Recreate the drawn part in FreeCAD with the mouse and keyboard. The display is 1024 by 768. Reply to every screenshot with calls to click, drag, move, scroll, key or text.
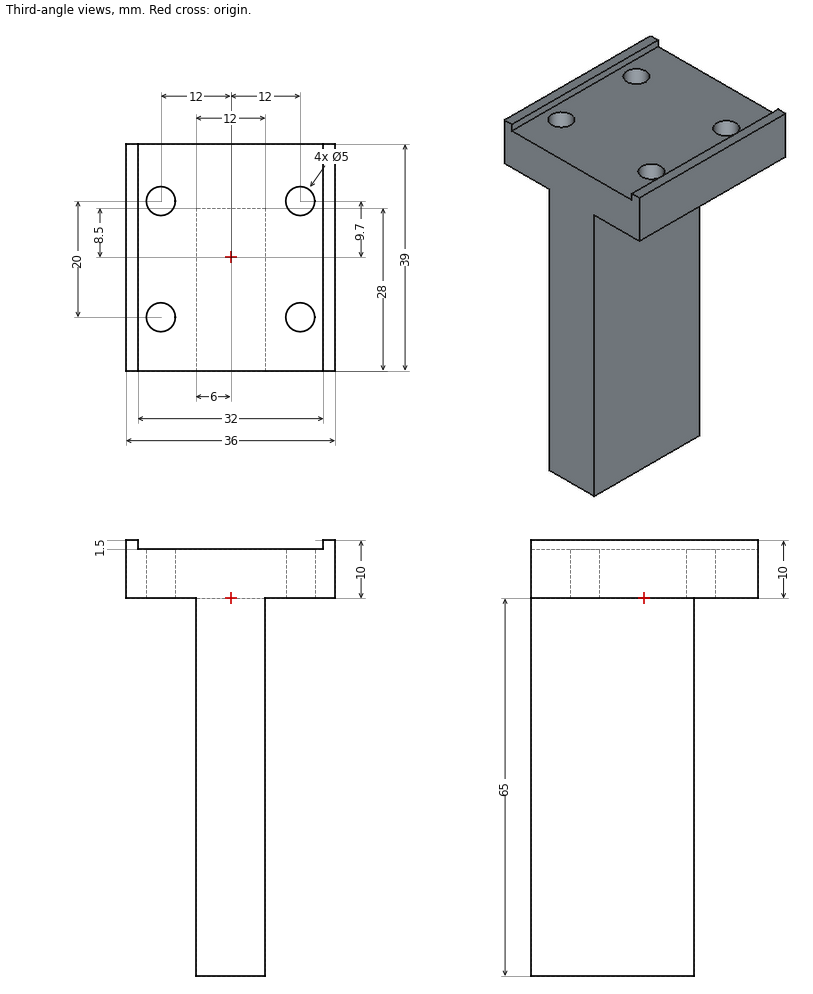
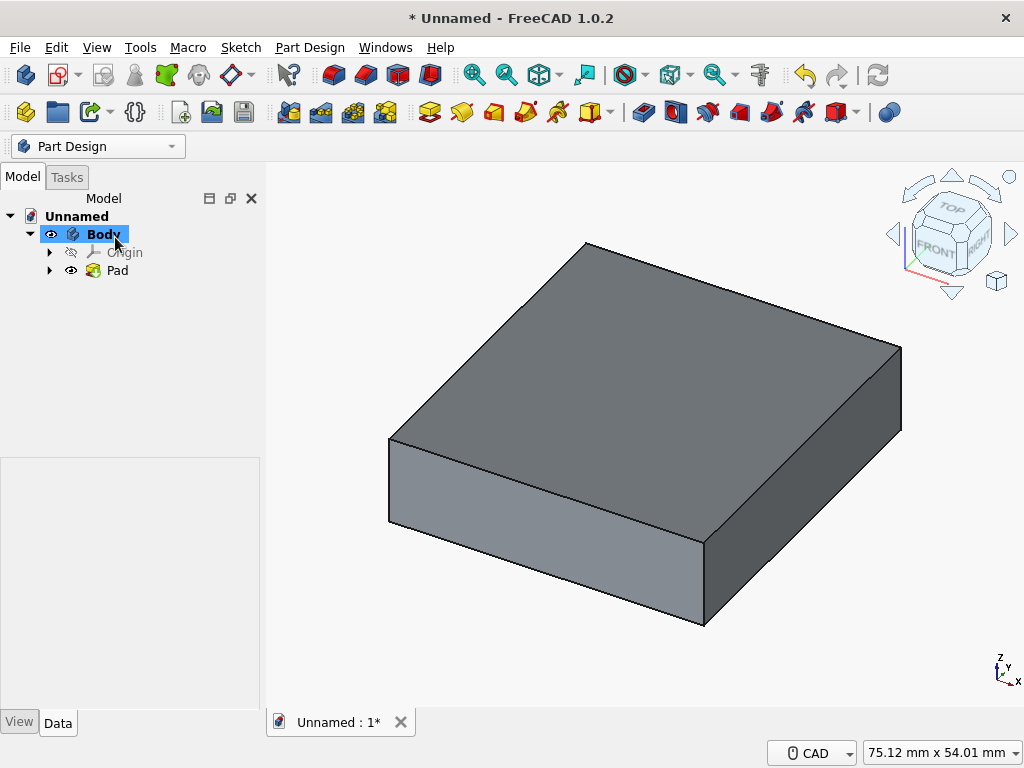
click(645, 392)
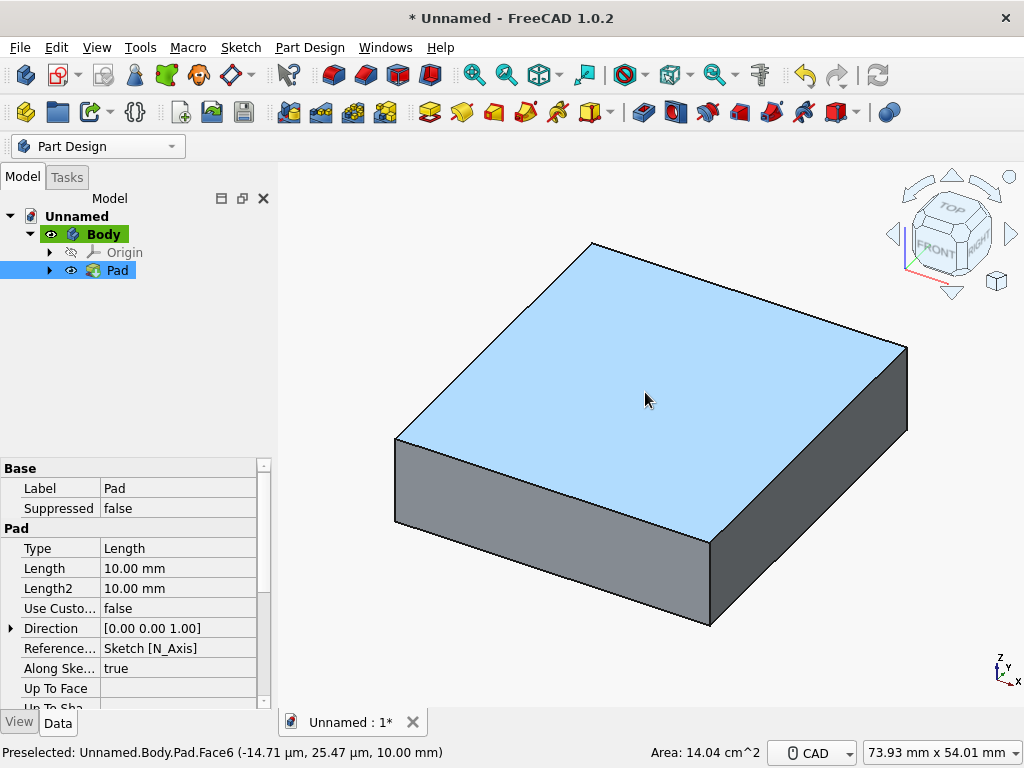
click(58, 76)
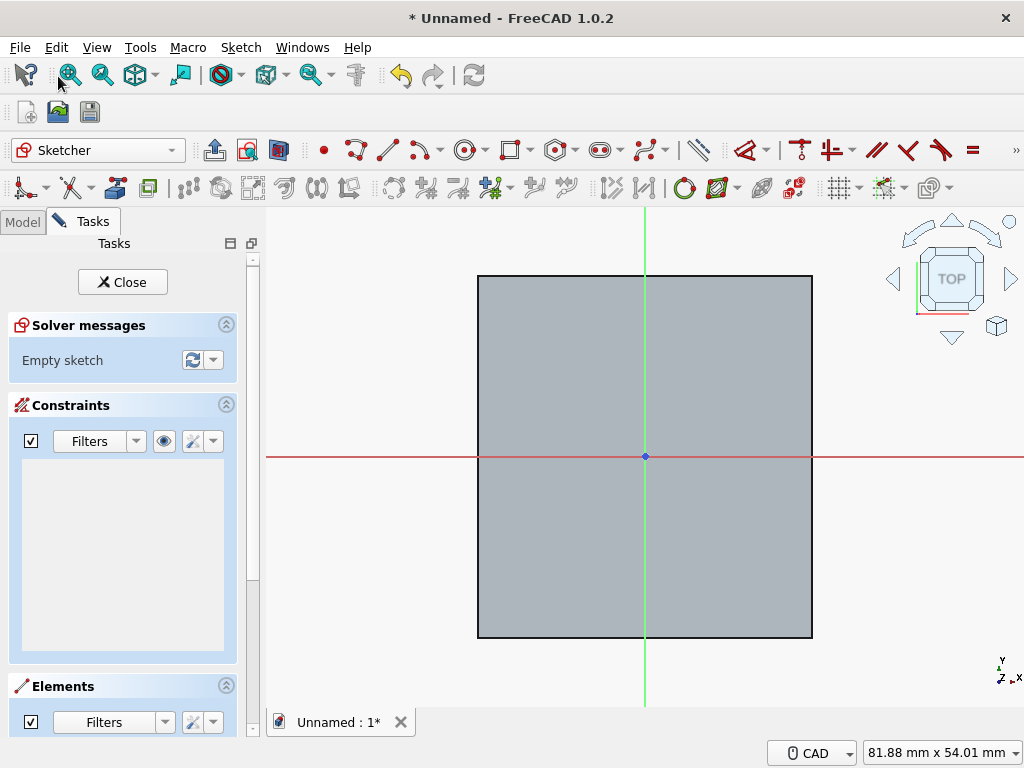
key(g)
key(v)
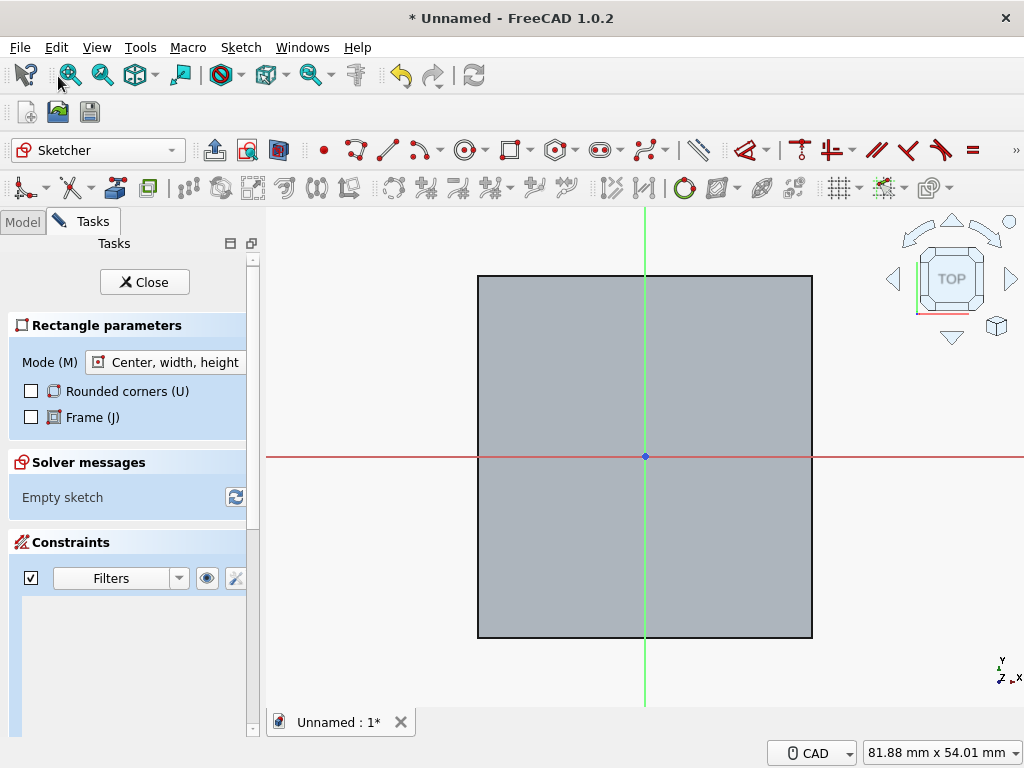
click(645, 457)
move(793, 276)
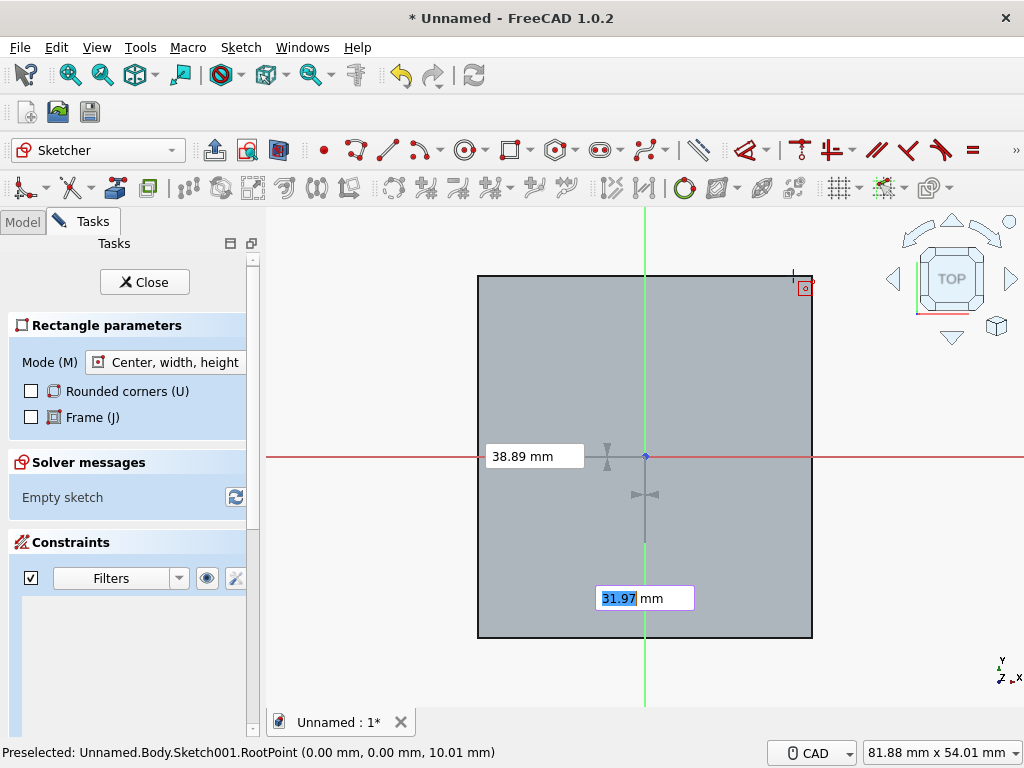
text(32)
key(Tab)
text(39)
key(Return)
key(Escape)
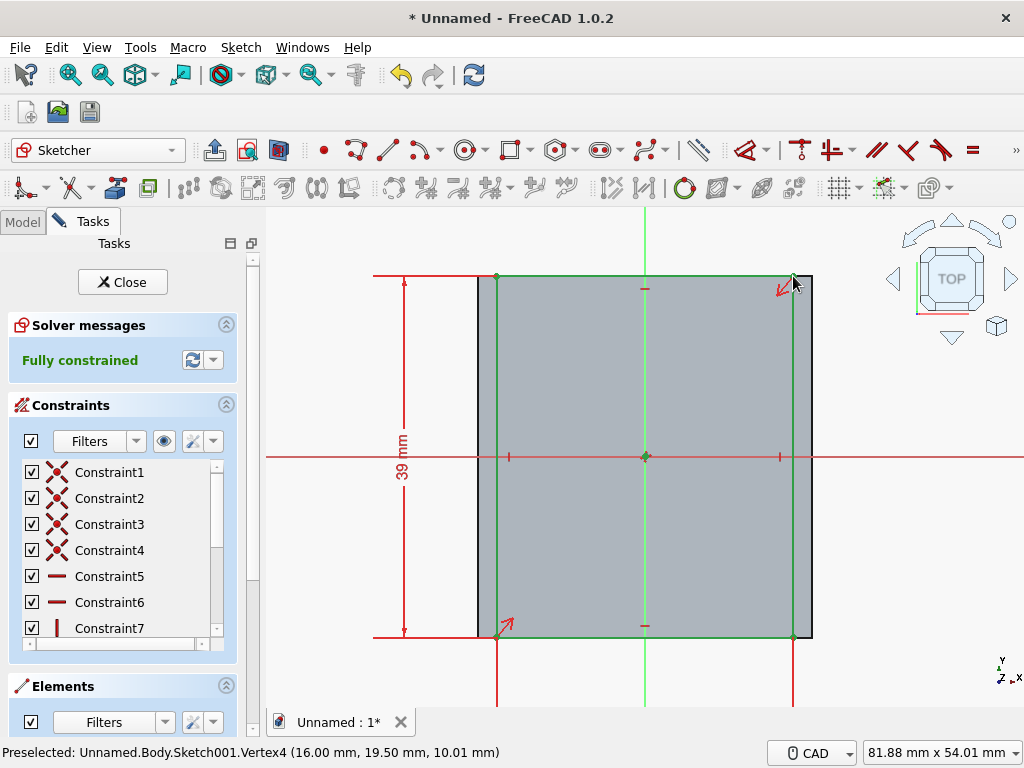
click(123, 282)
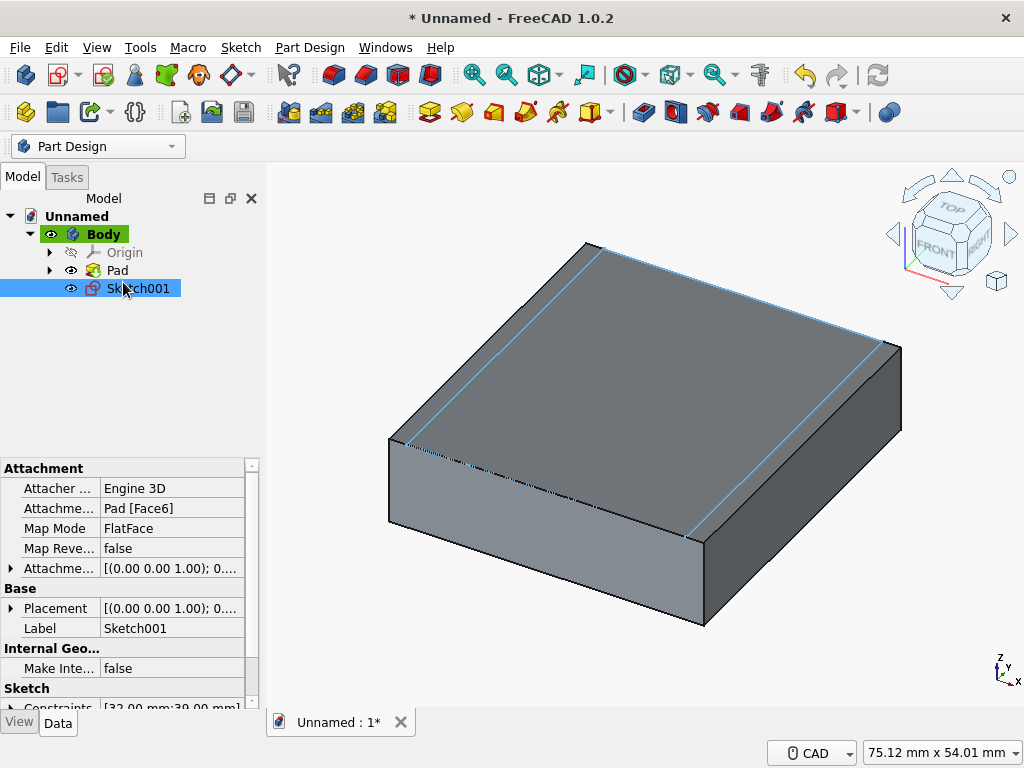
click(644, 112)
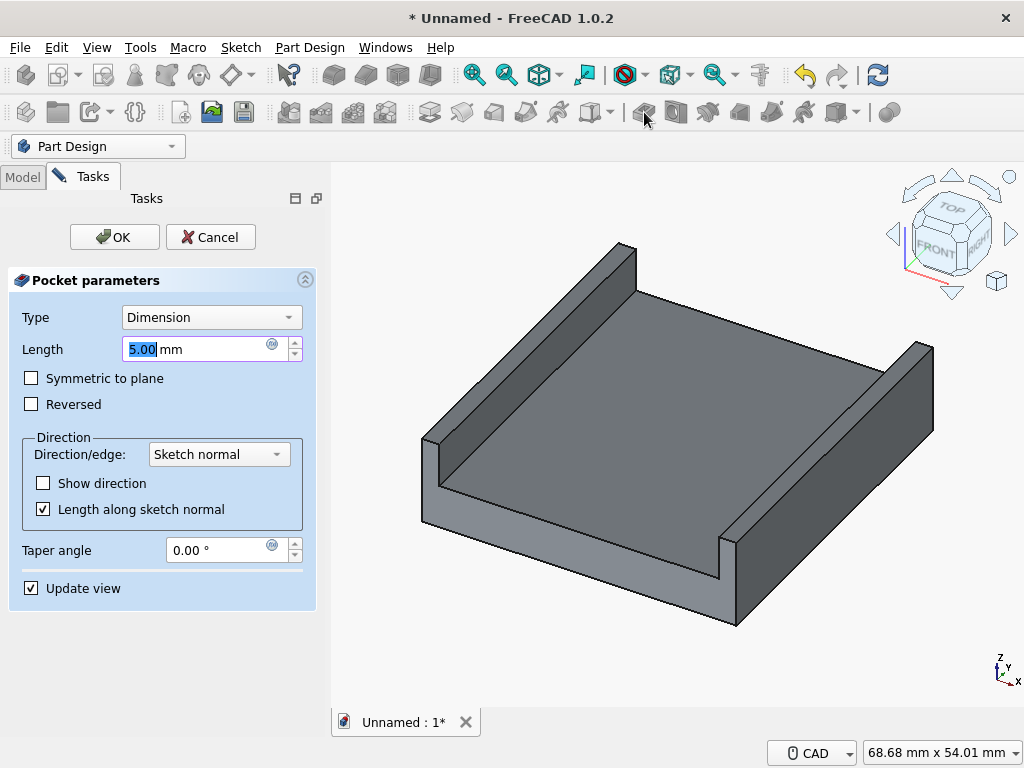
text(1.5)
key(Tab)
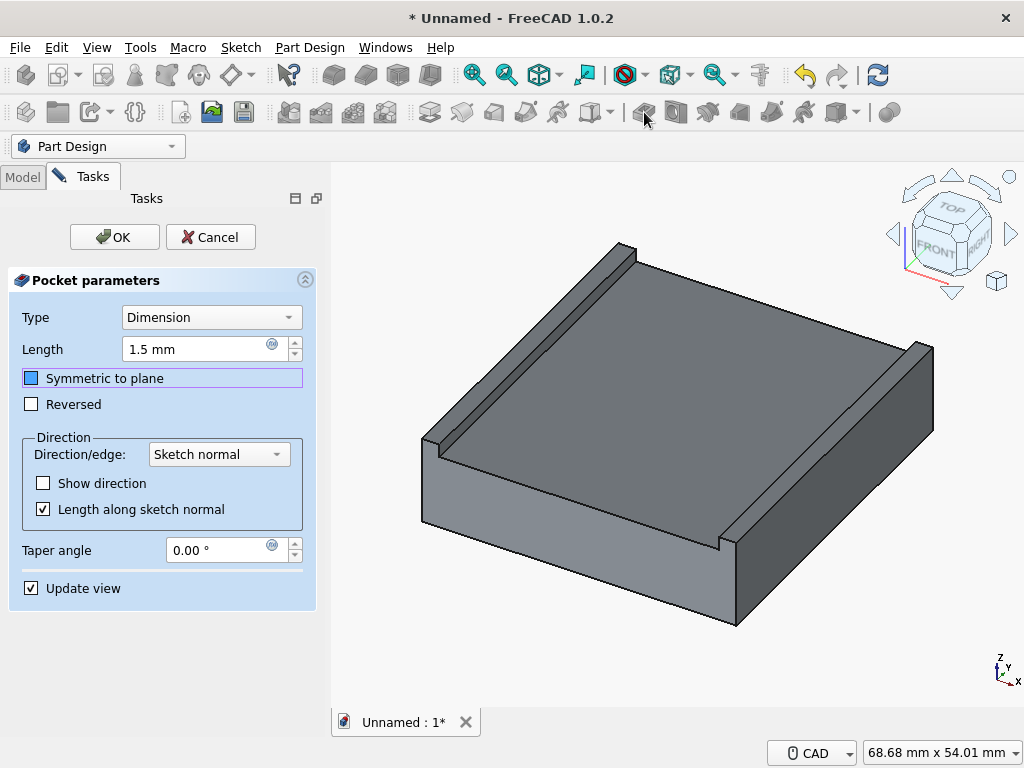
click(115, 237)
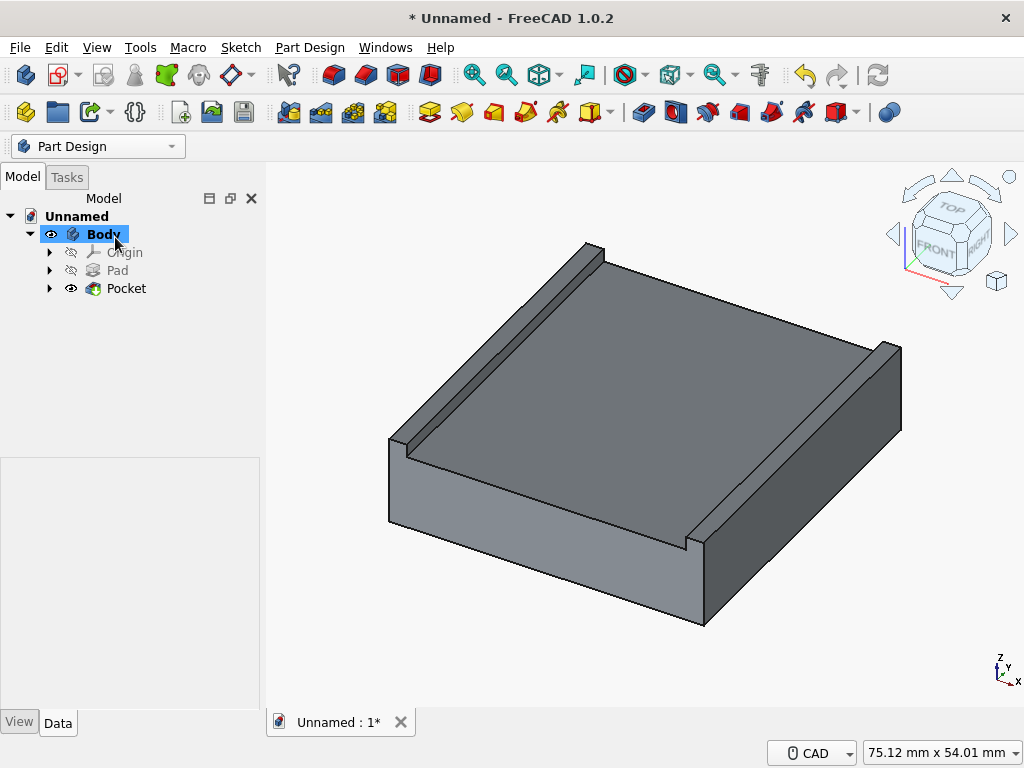
key(5)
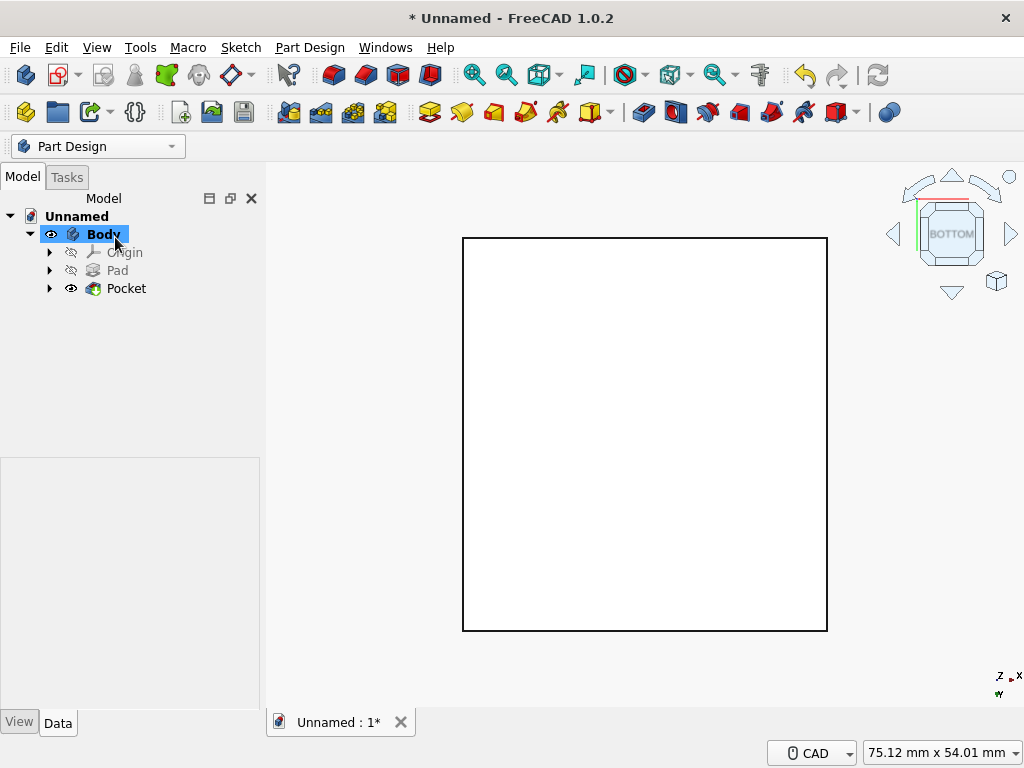
click(645, 433)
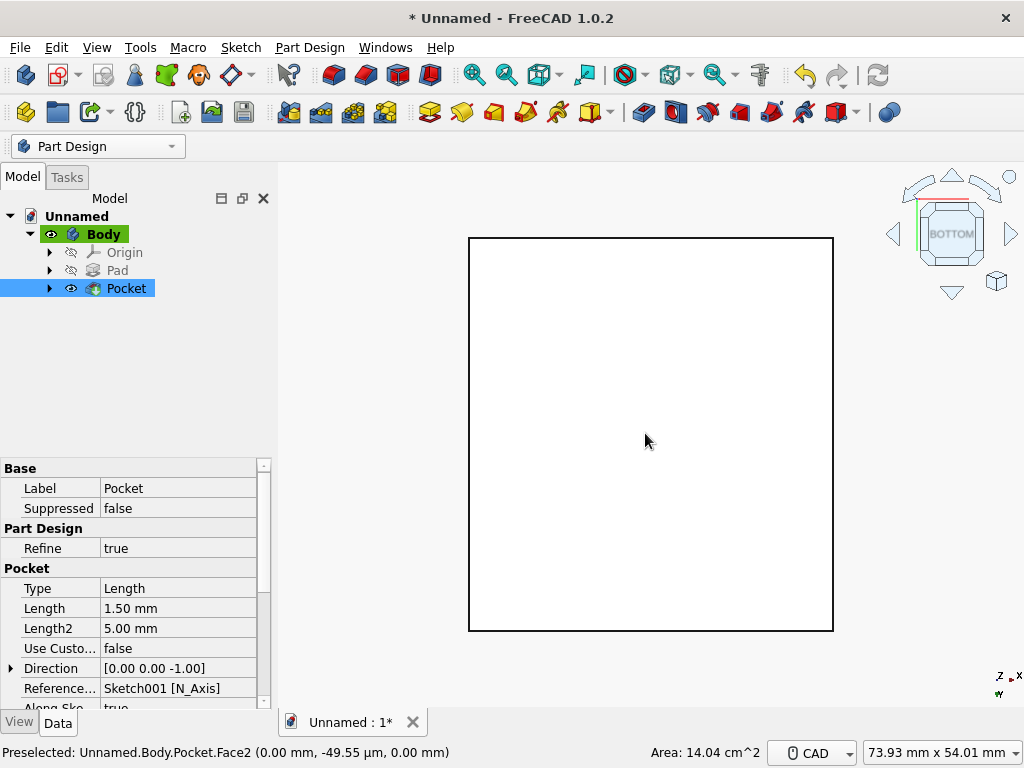
click(58, 76)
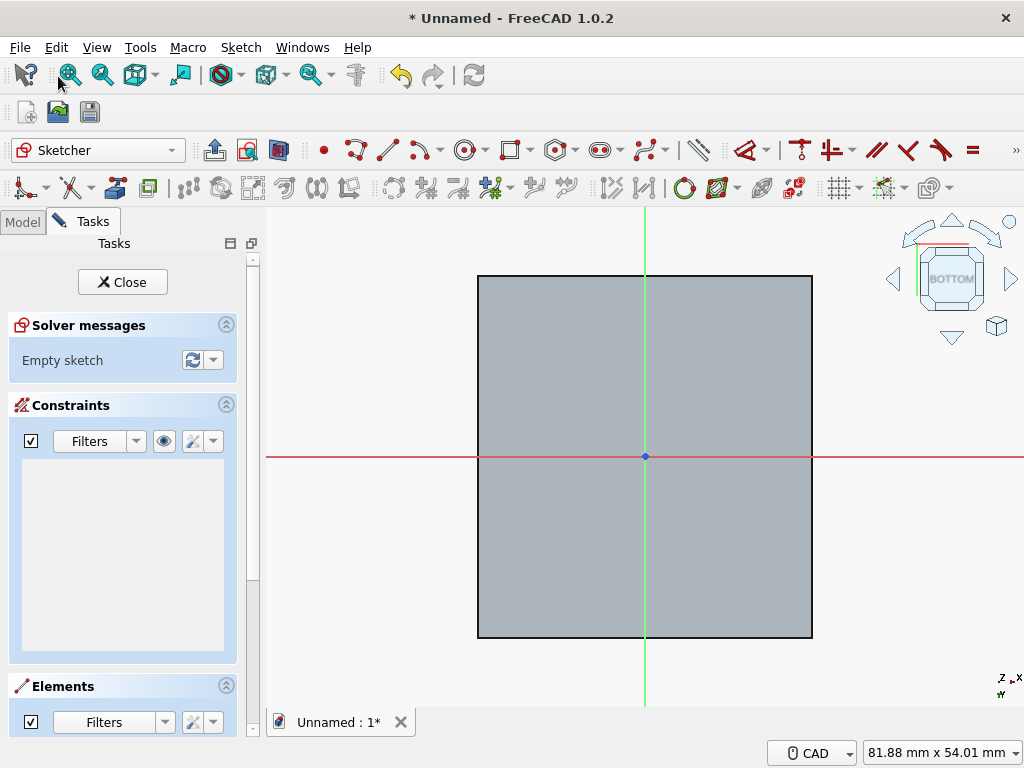
click(510, 150)